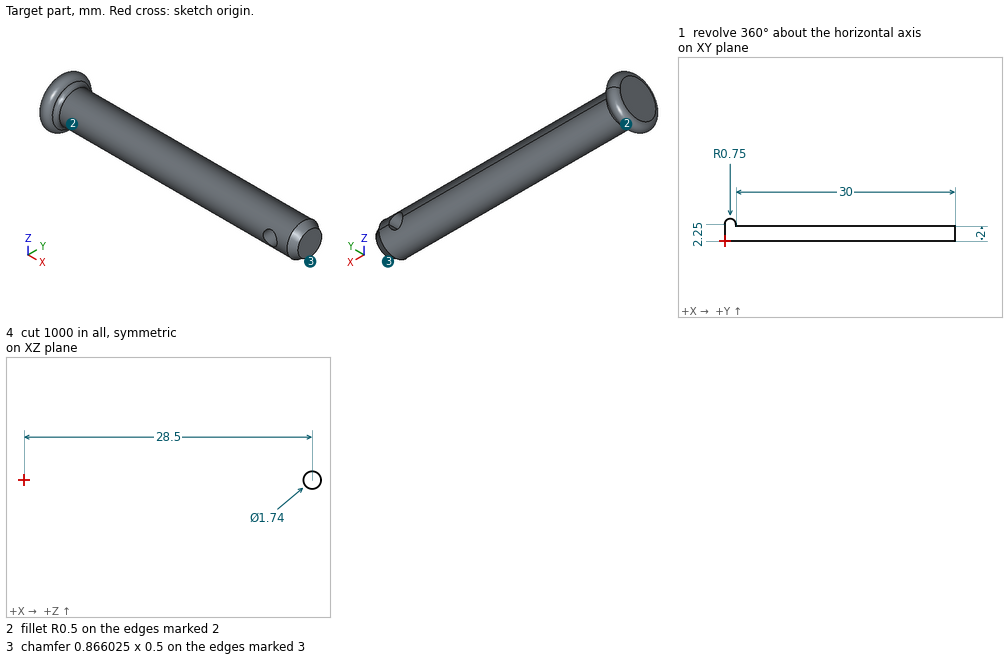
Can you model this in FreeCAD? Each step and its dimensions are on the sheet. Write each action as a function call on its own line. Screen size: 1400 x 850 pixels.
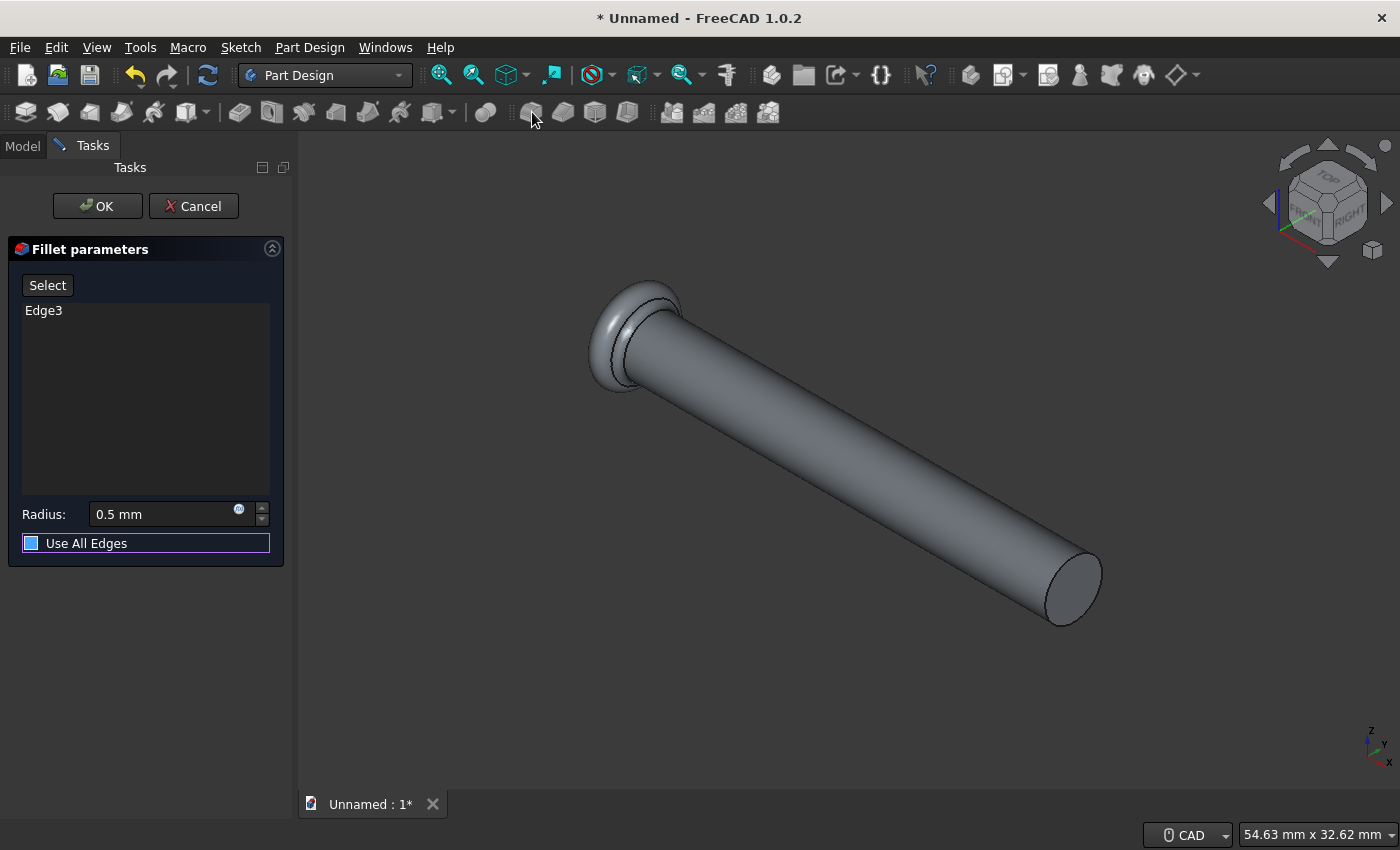
click(98, 206)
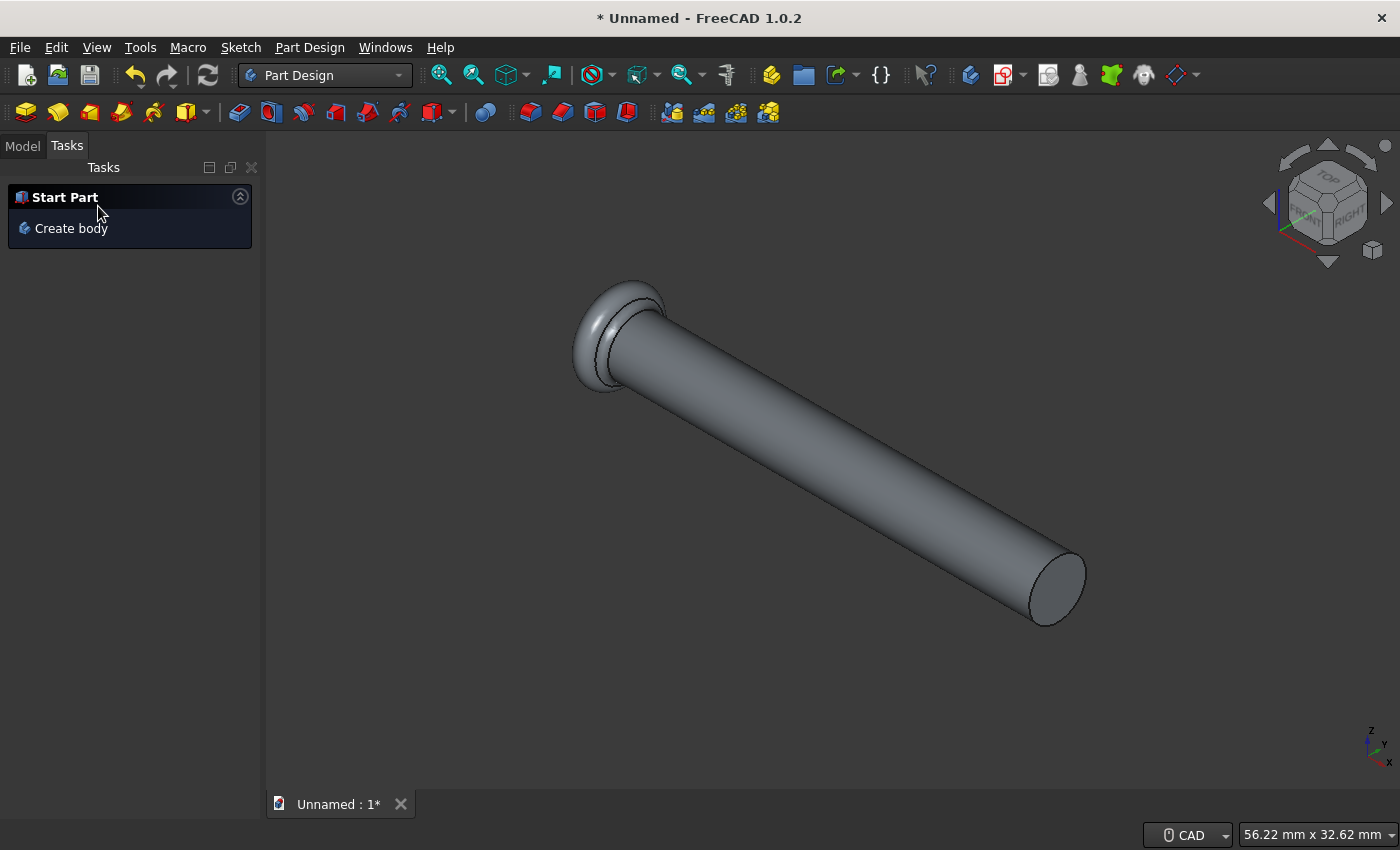
click(1029, 605)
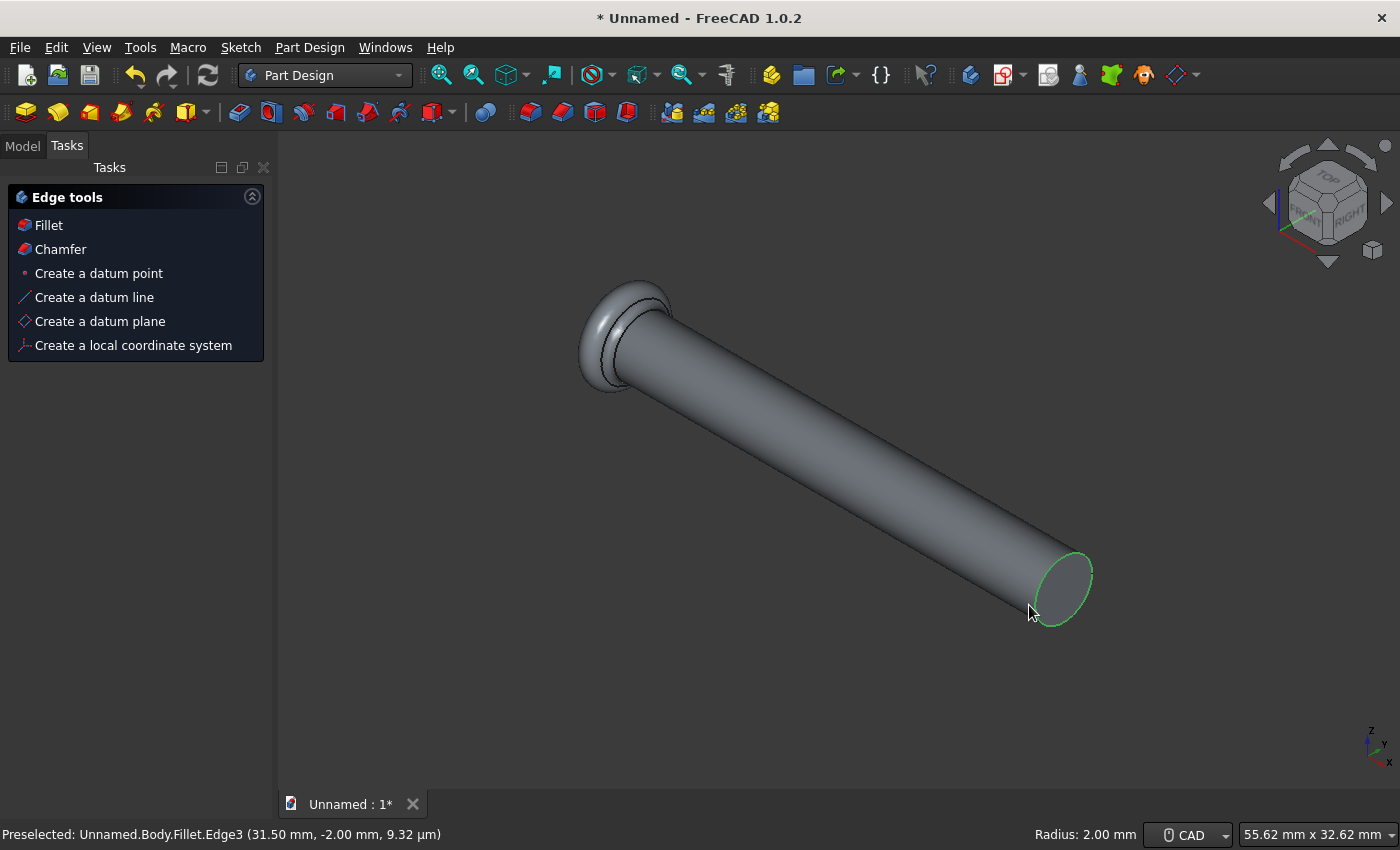
click(564, 112)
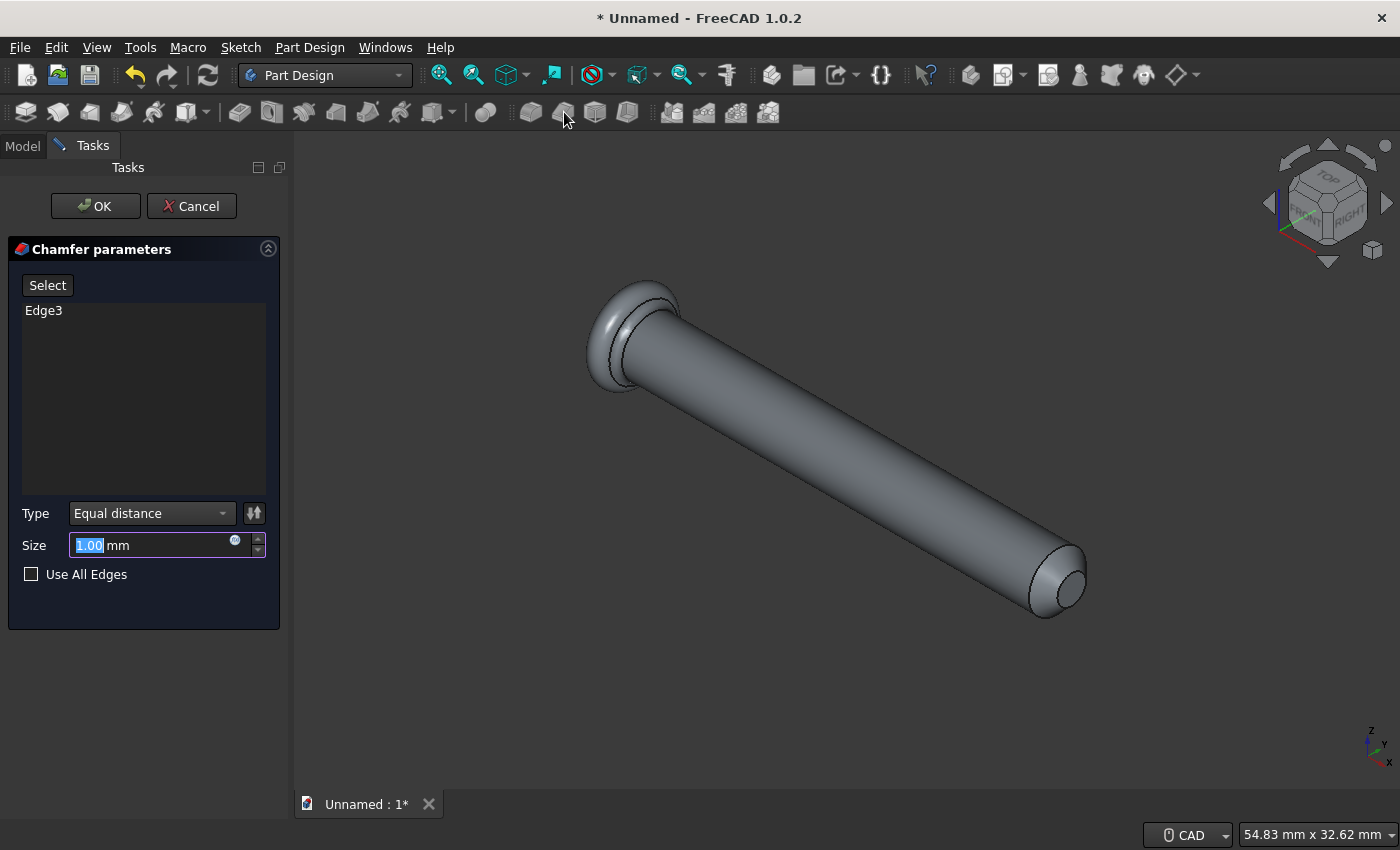
text(0.866025)
key(Tab)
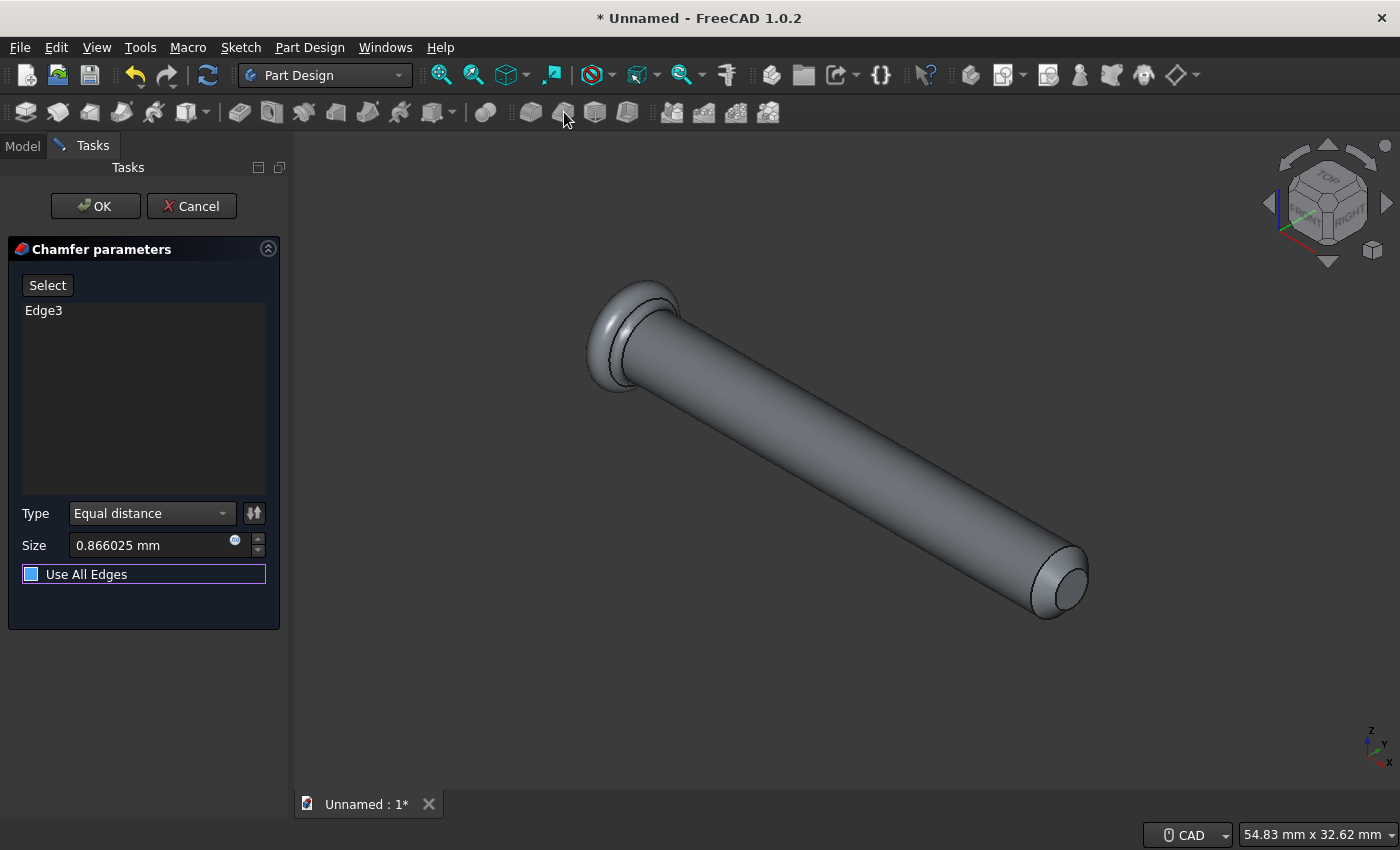
click(153, 514)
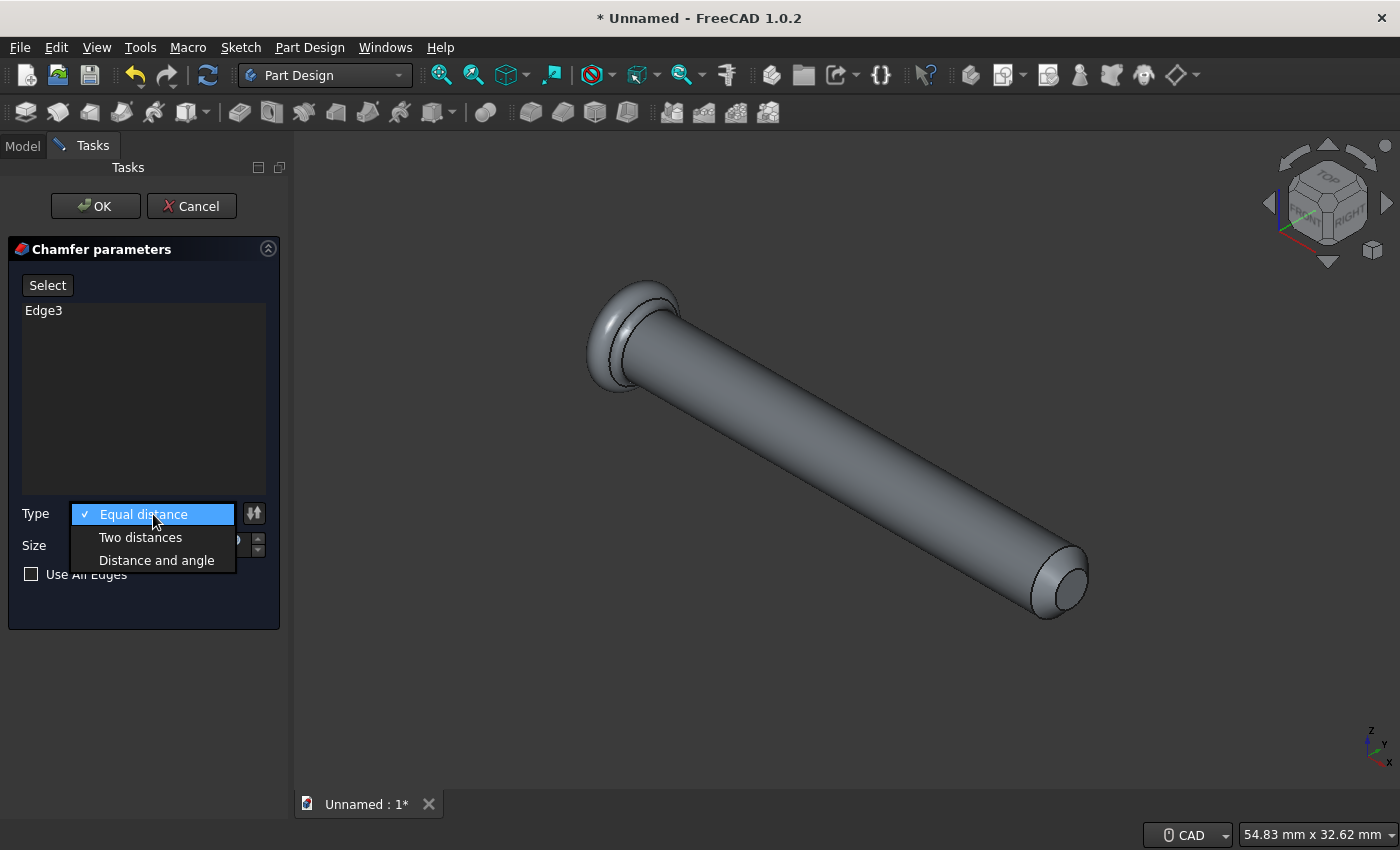
click(152, 538)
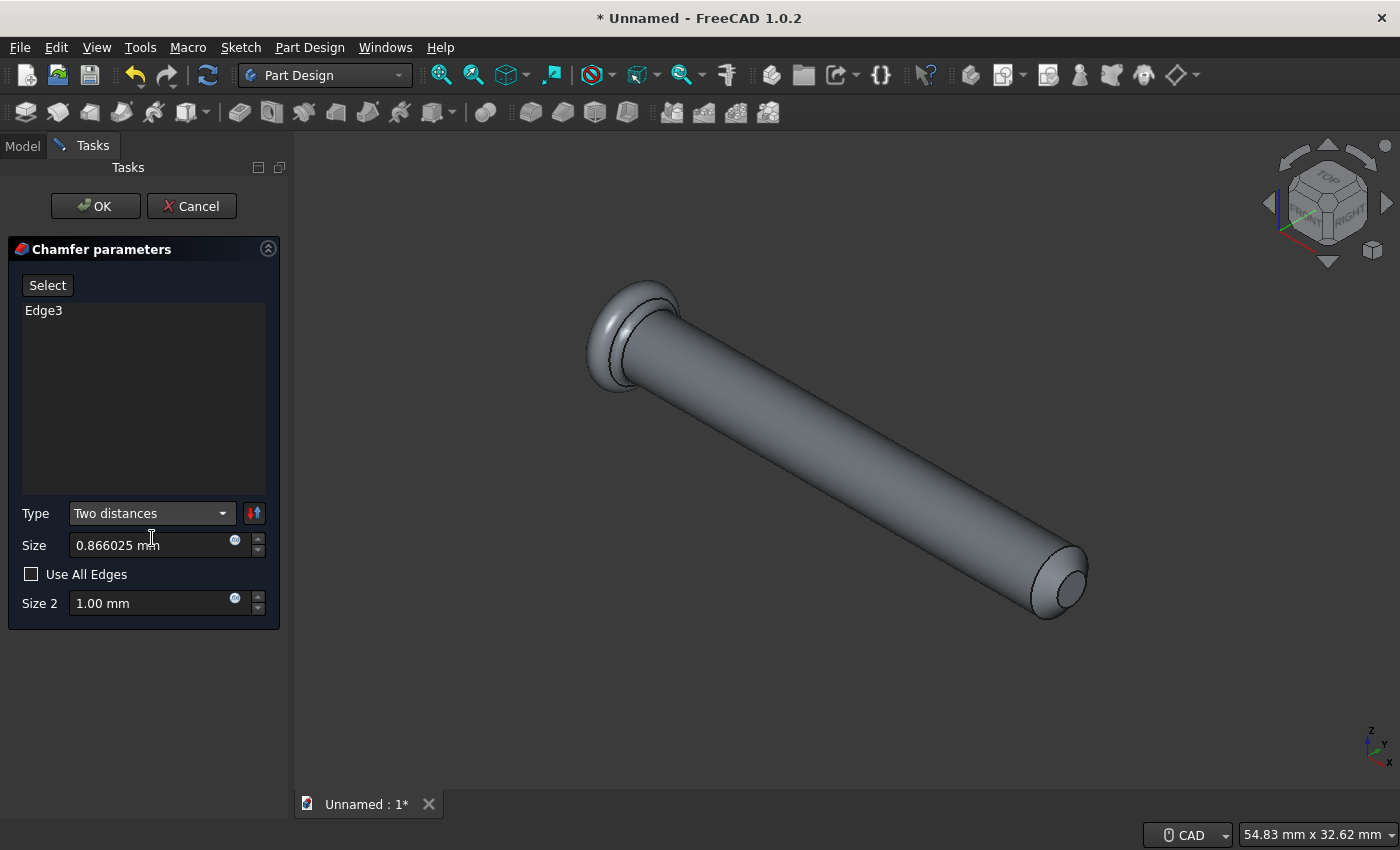
triple_click(160, 603)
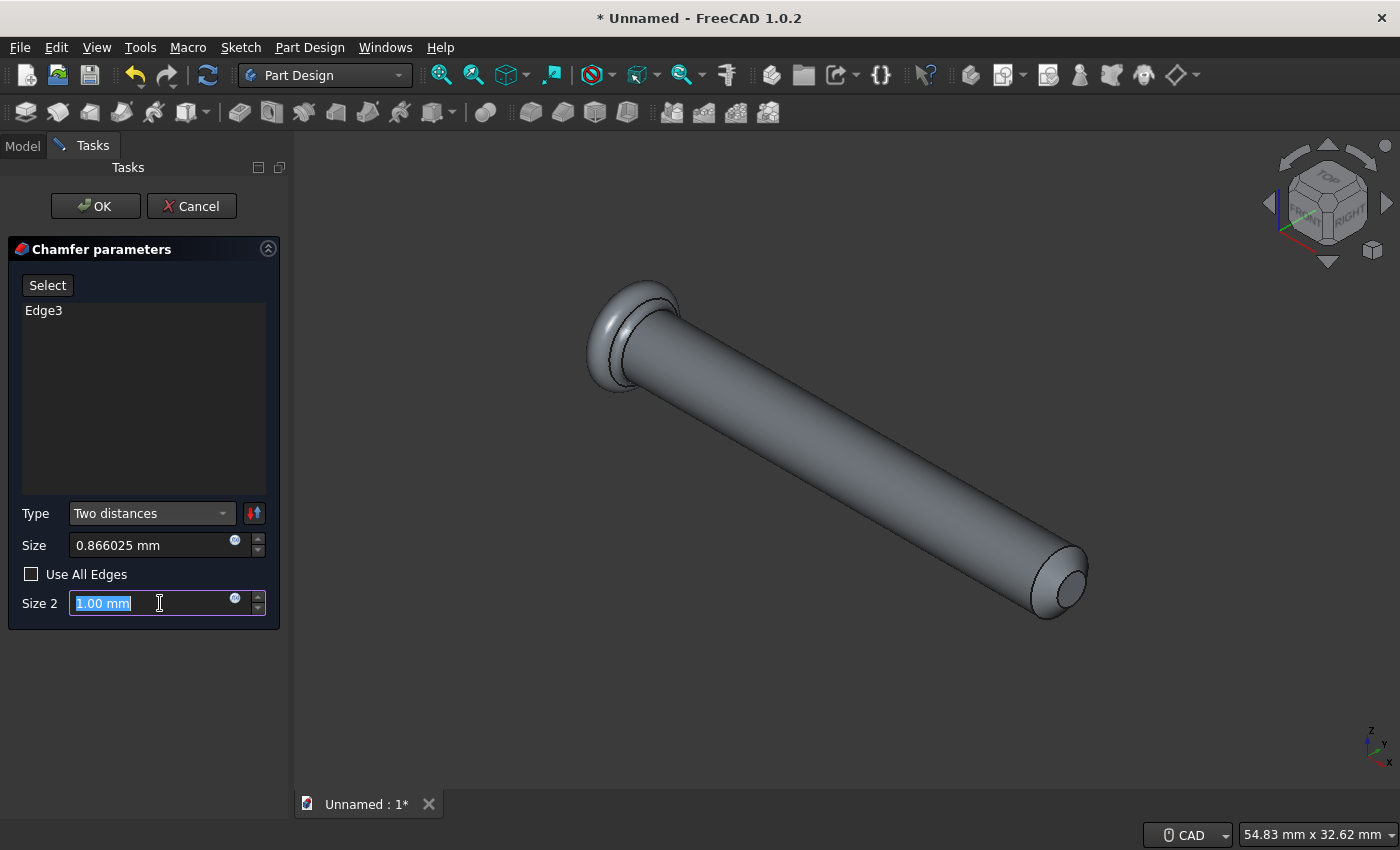
text(0.5)
key(Tab)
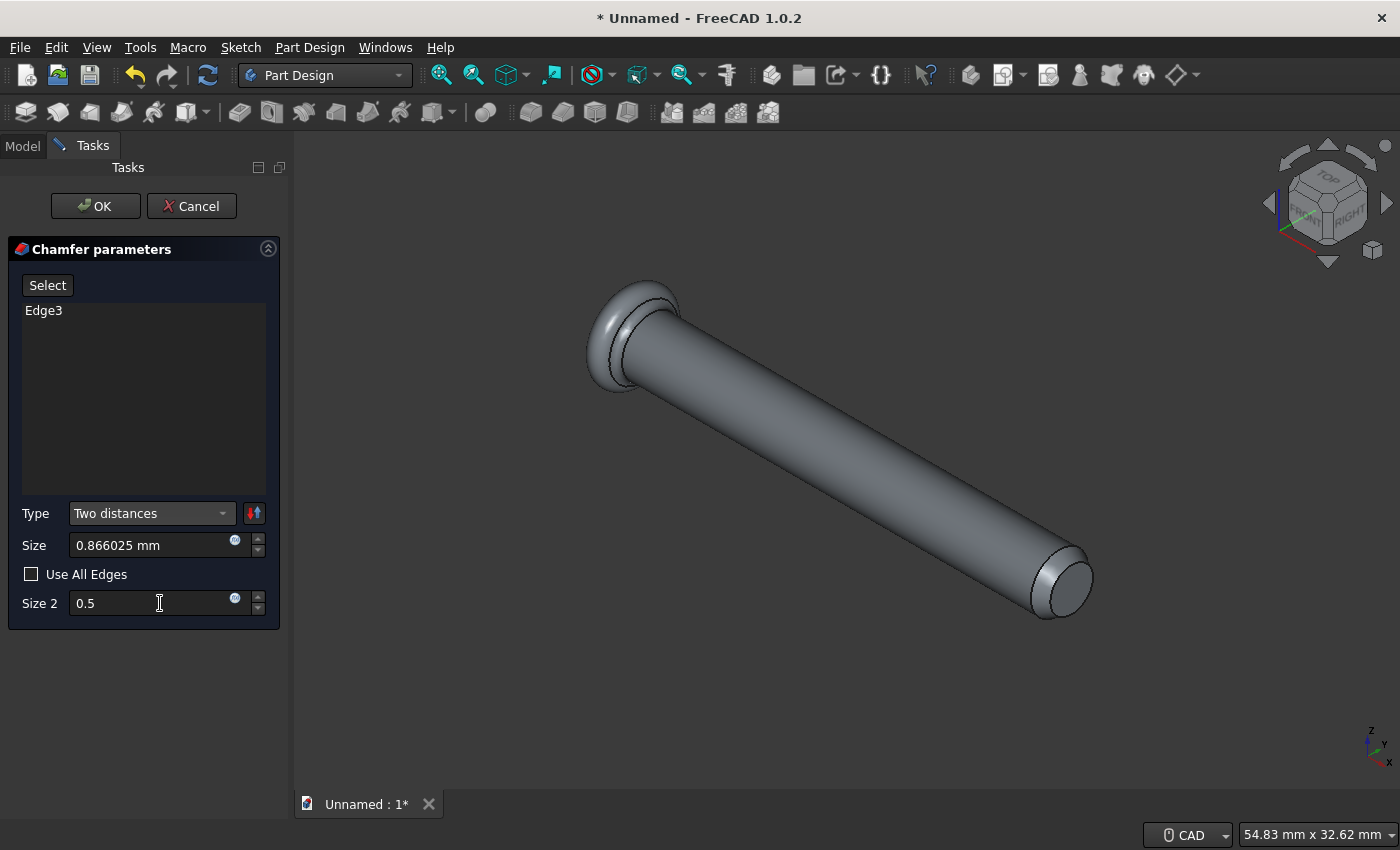
click(96, 206)